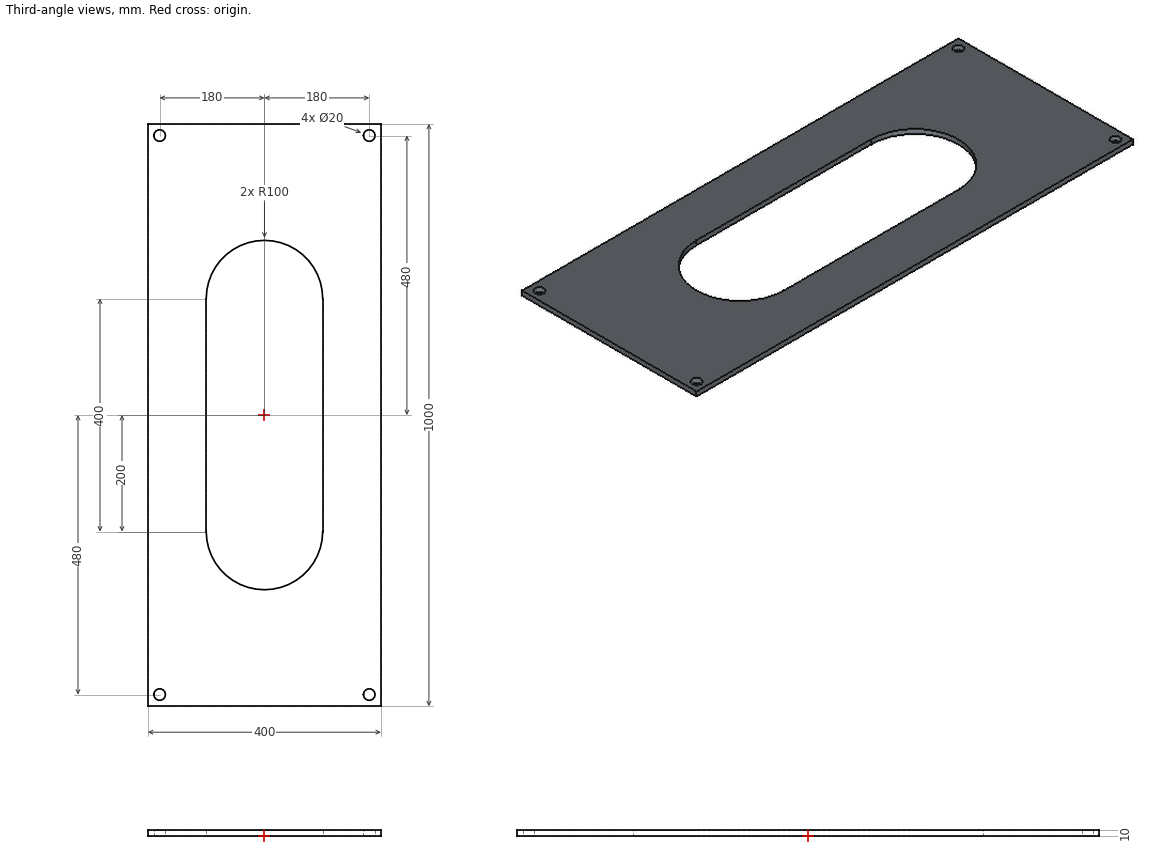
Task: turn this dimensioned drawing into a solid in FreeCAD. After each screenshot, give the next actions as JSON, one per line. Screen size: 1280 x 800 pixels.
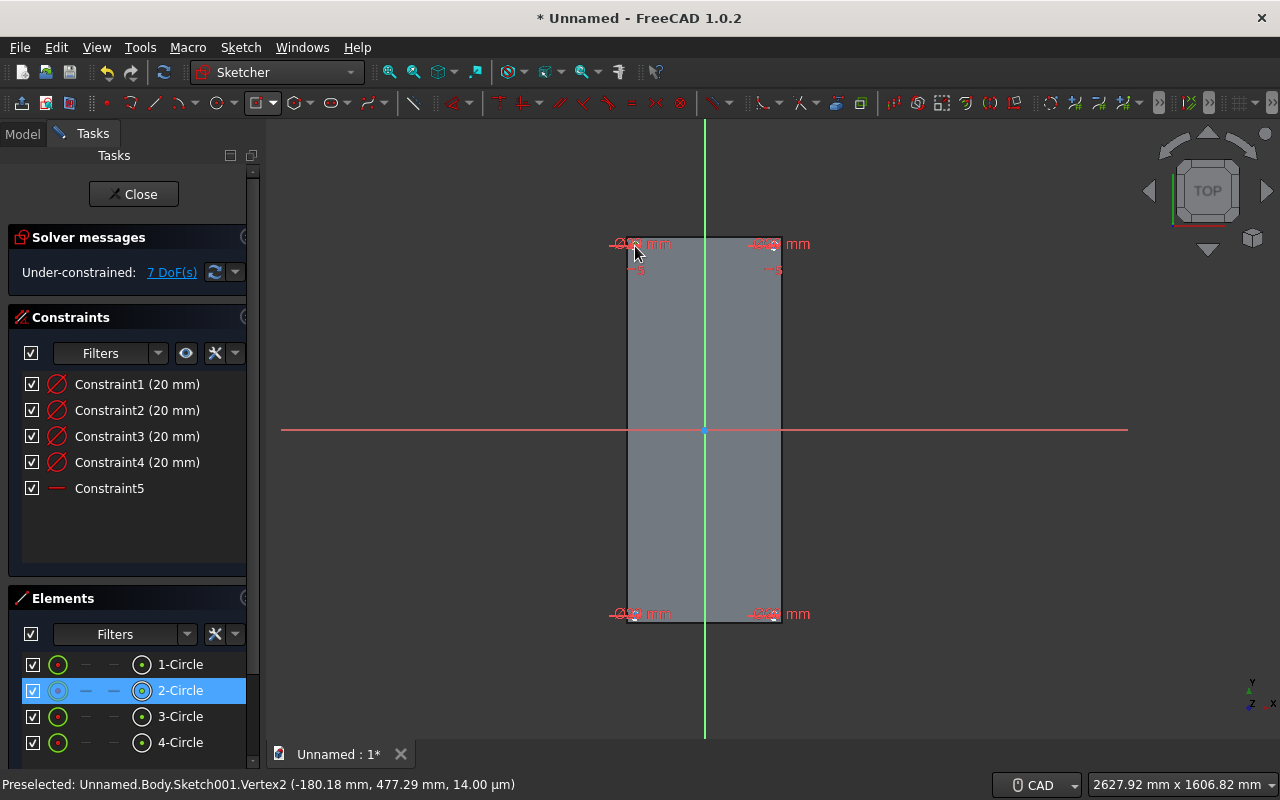
{"action": "left_click", "coordinate": [635, 616]}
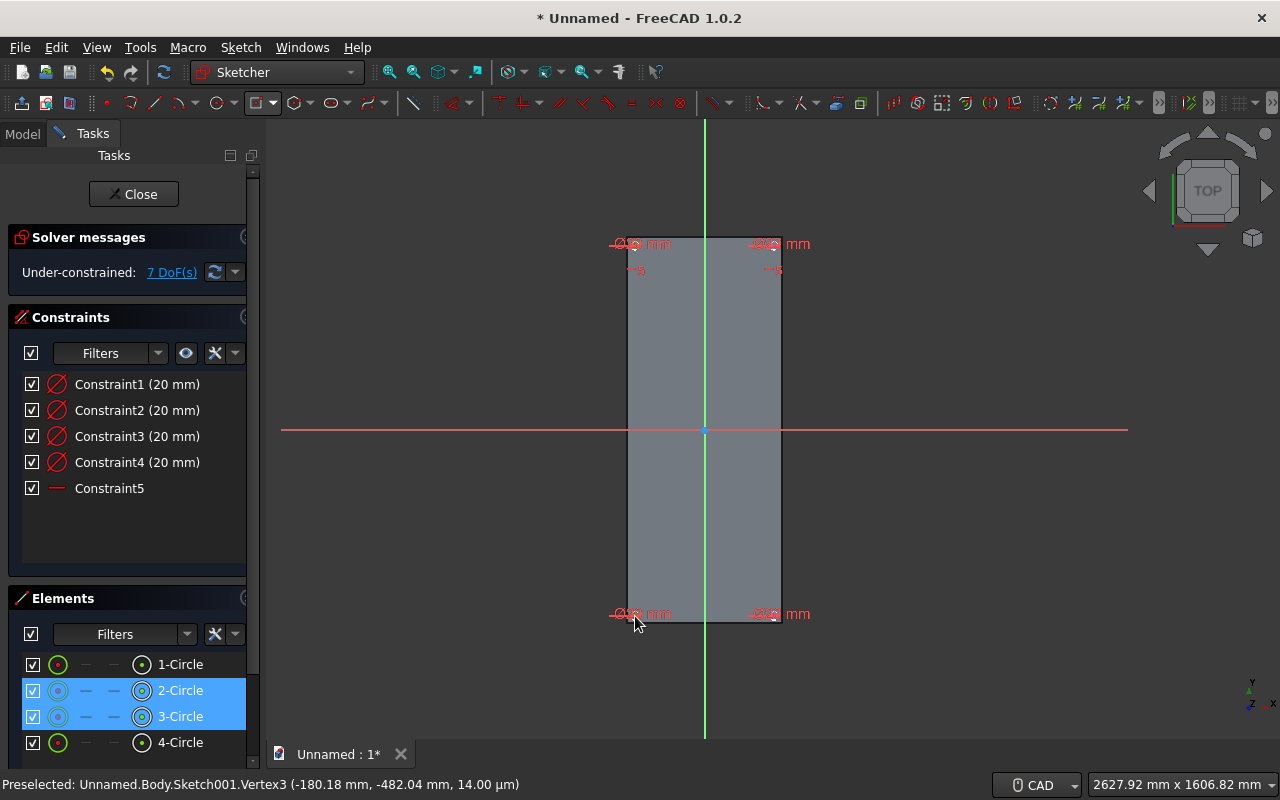
{"action": "left_click", "coordinate": [542, 104]}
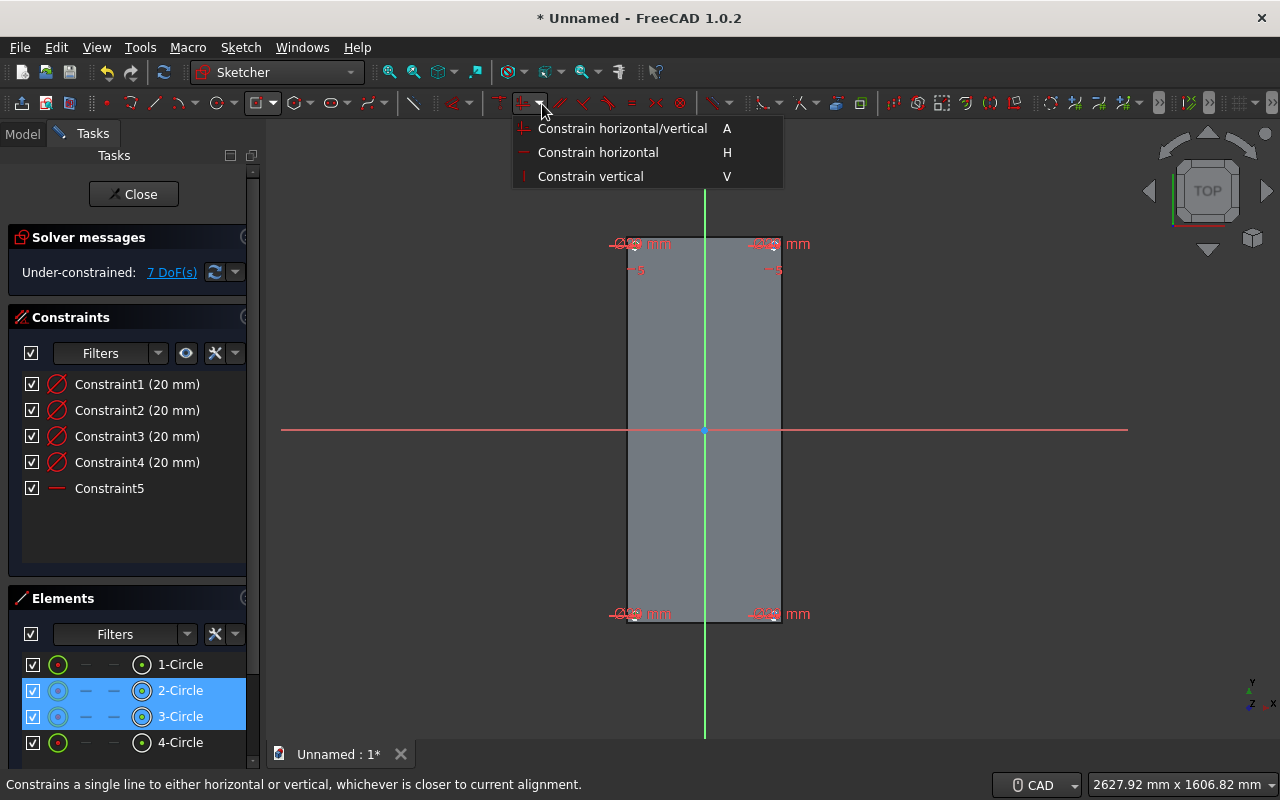
{"action": "left_click", "coordinate": [648, 176]}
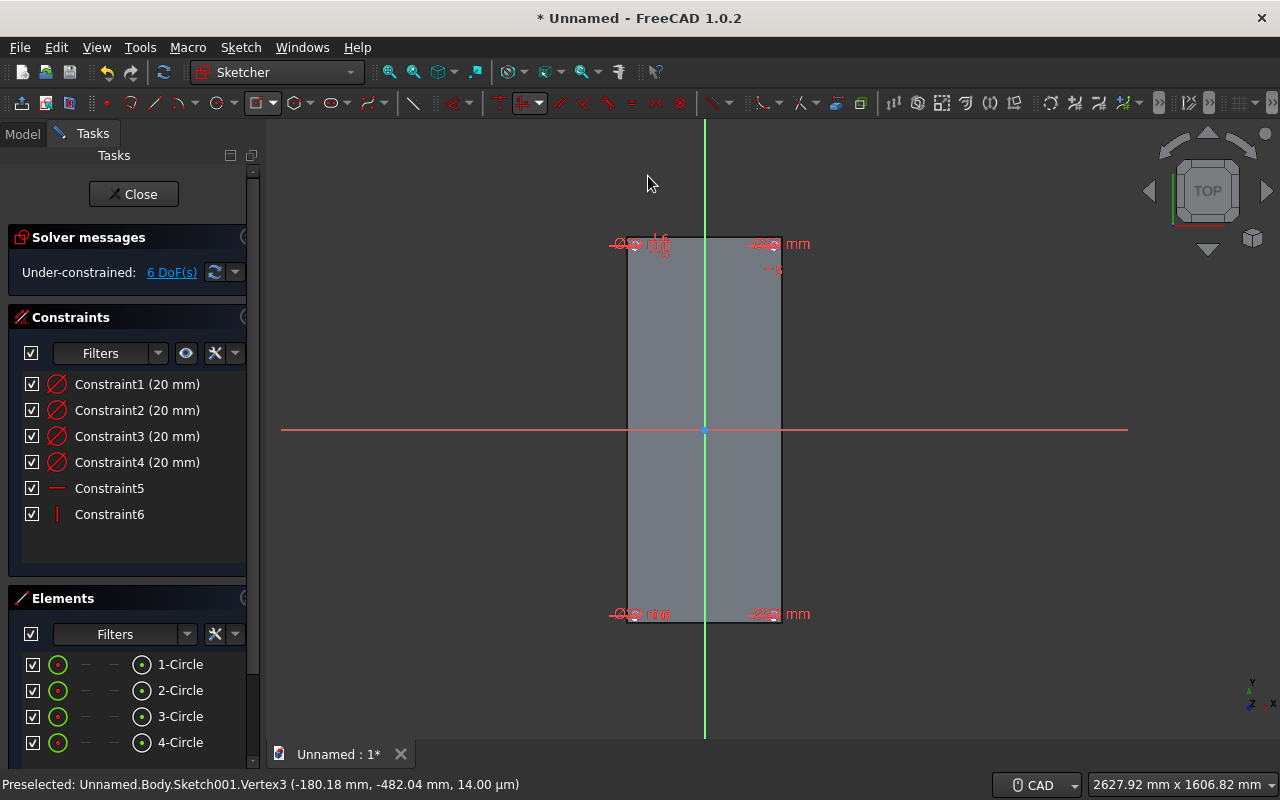
{"action": "left_click", "coordinate": [774, 246]}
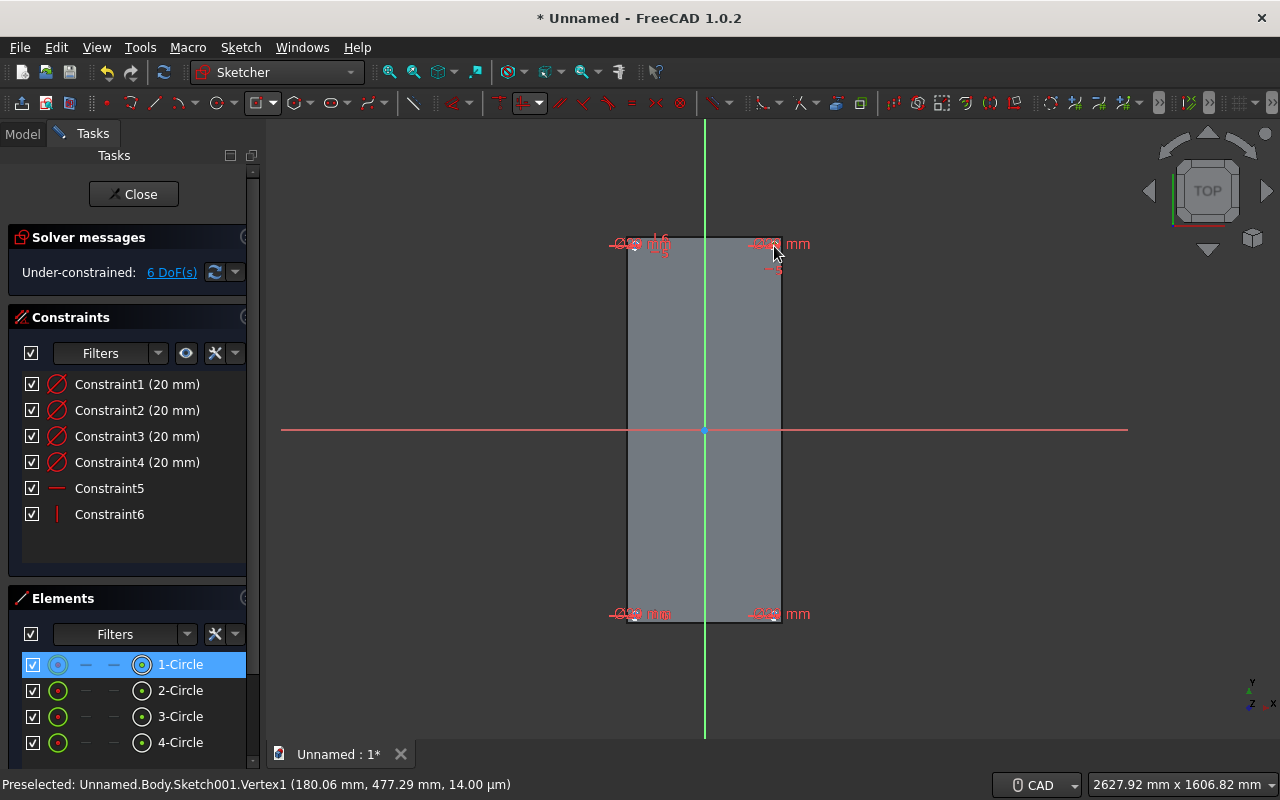
{"action": "left_click", "coordinate": [774, 616]}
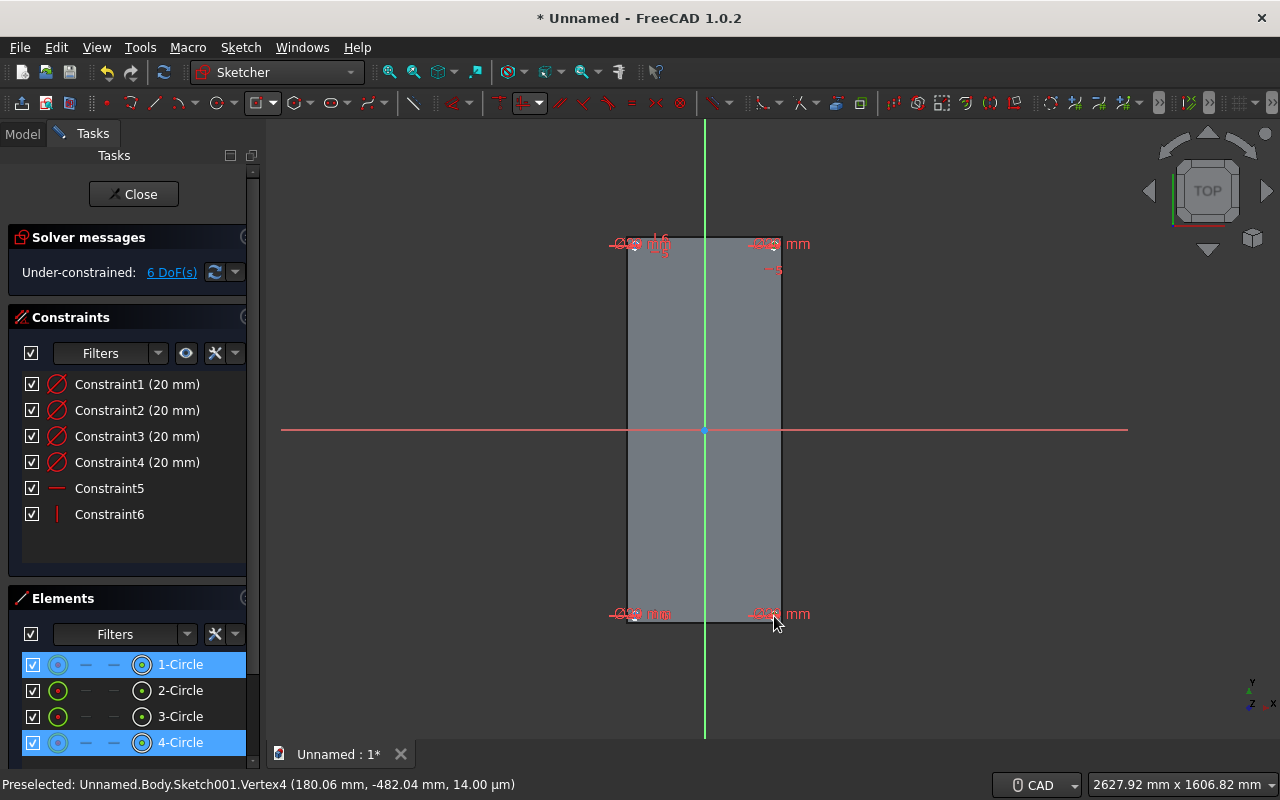
{"action": "key", "text": "v"}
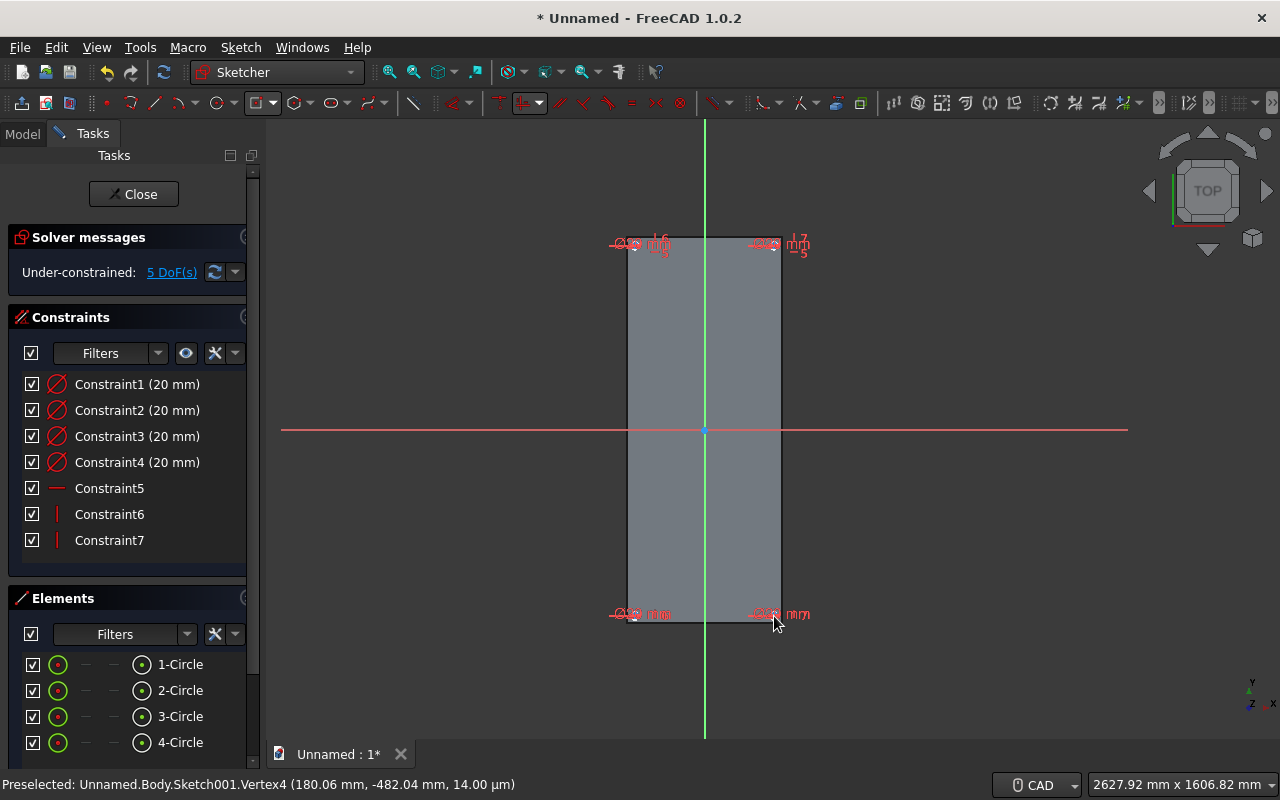
{"action": "left_click", "coordinate": [635, 616]}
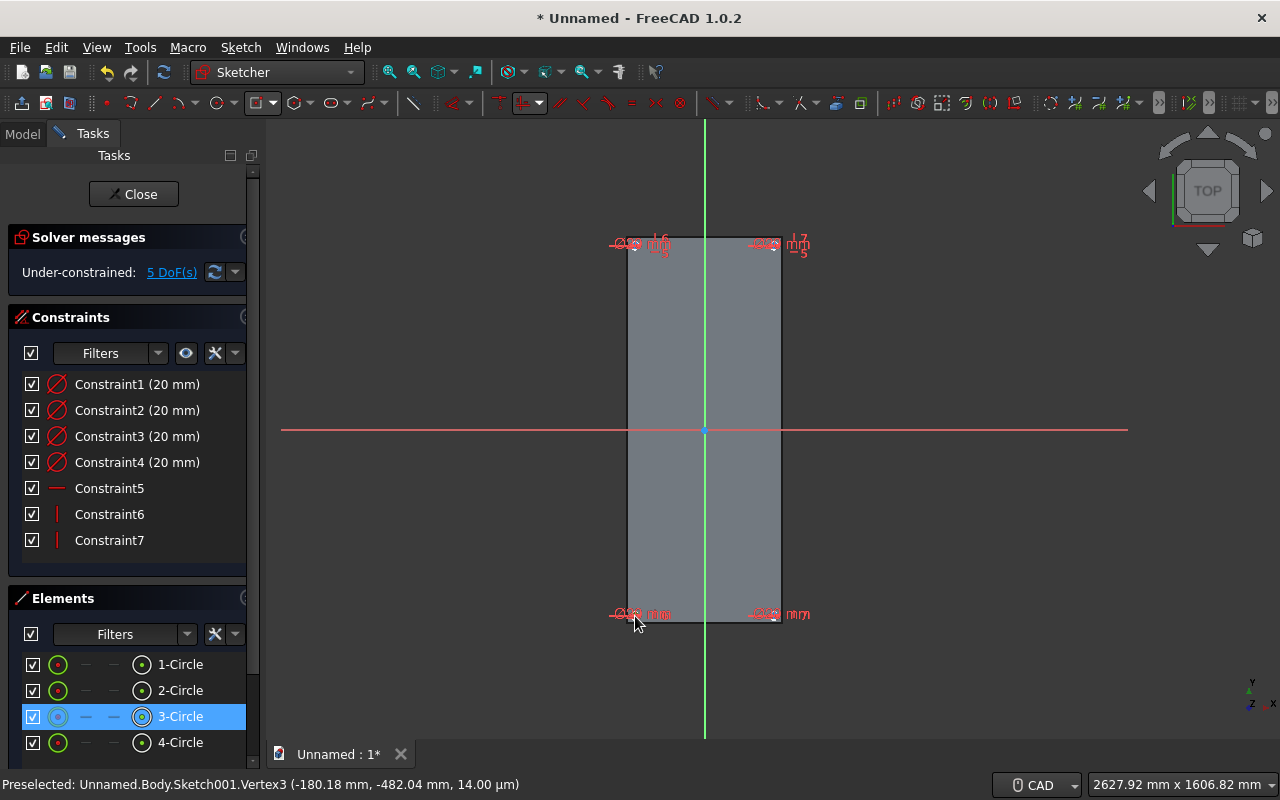
{"action": "left_click", "coordinate": [774, 616]}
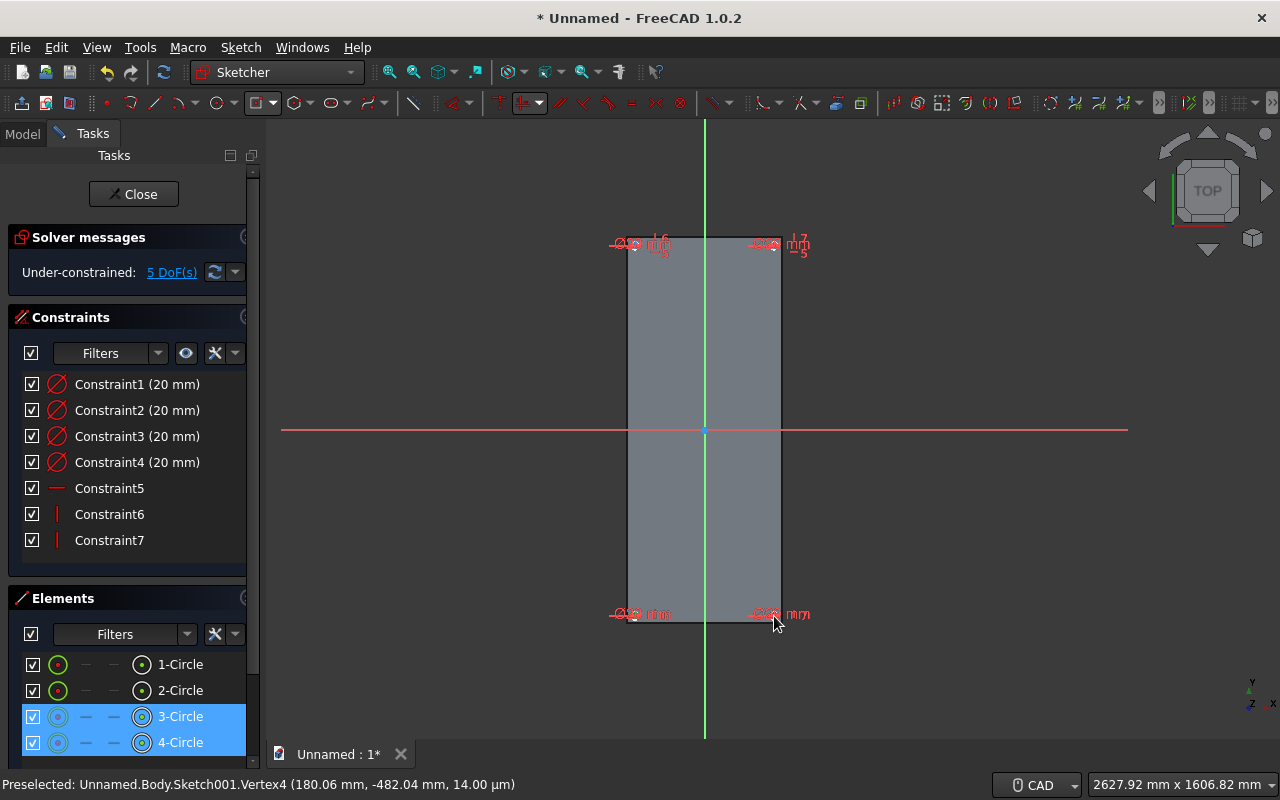
{"action": "left_click", "coordinate": [542, 104]}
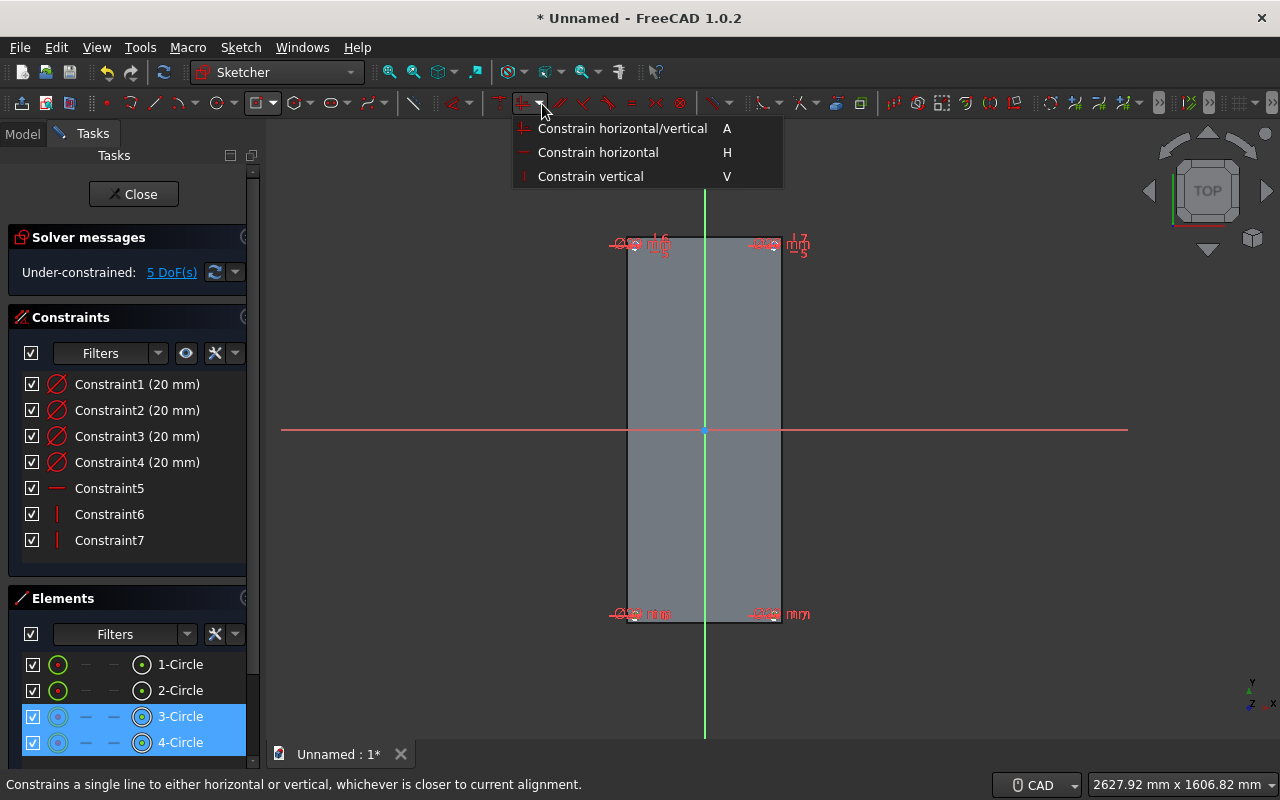
{"action": "left_click", "coordinate": [648, 152]}